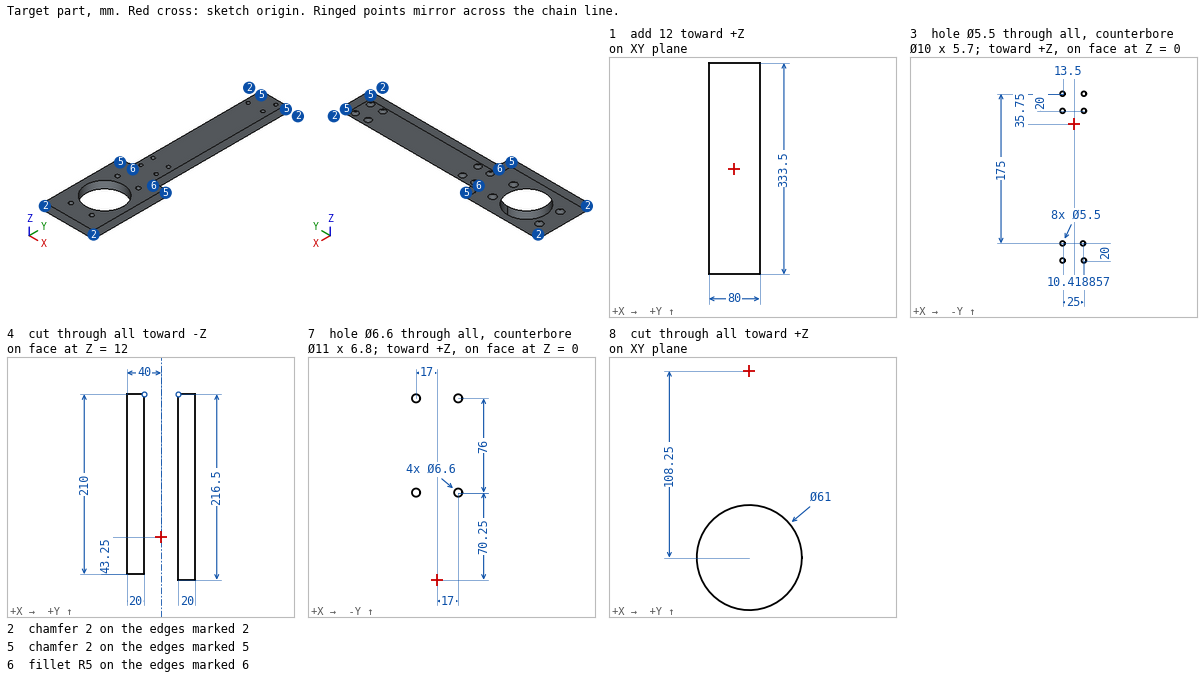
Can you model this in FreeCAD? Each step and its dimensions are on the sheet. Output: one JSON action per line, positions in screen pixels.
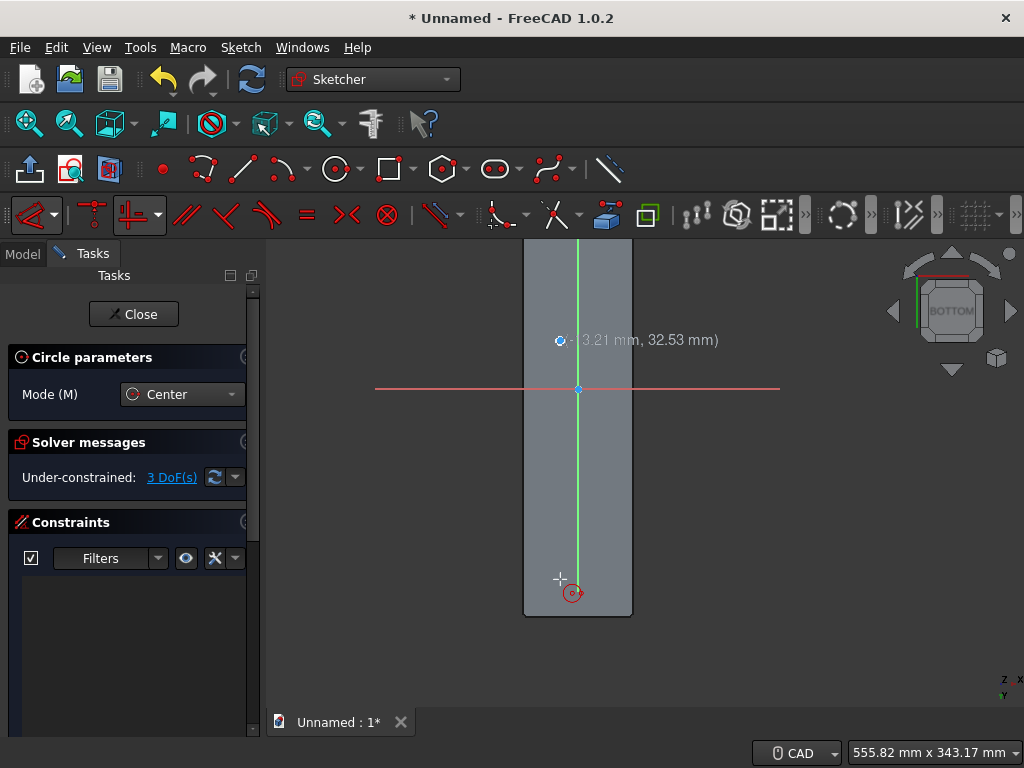
{"action": "left_click", "coordinate": [560, 579]}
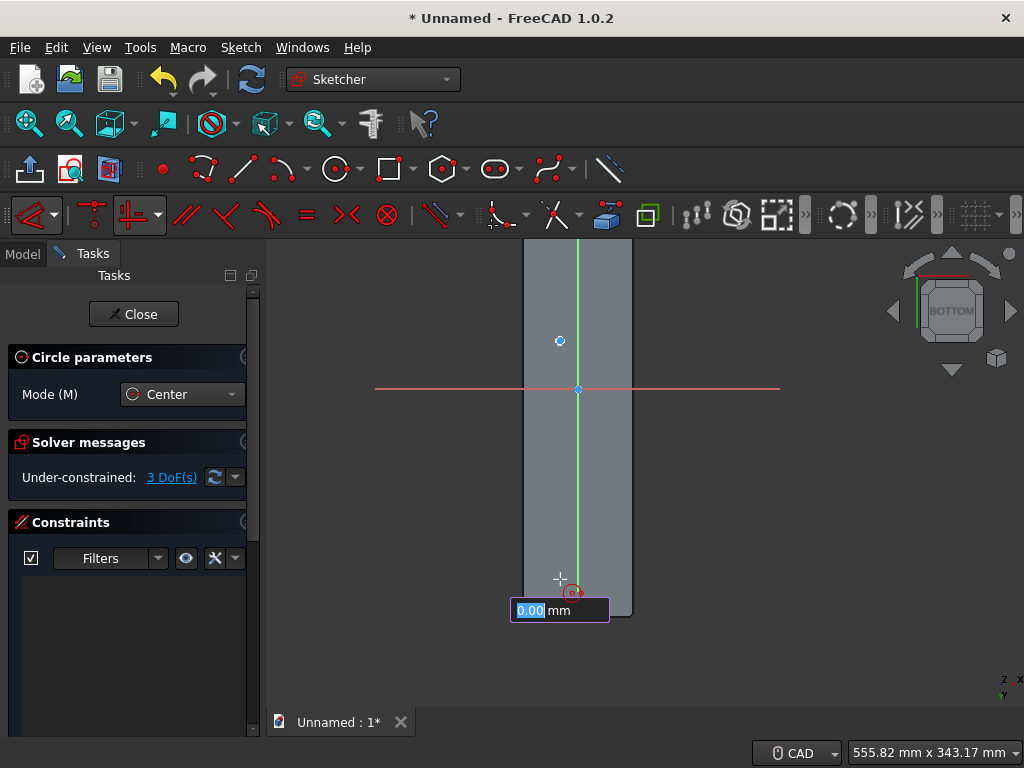
{"action": "scroll", "coordinate": [562, 576], "scroll_direction": "up", "scroll_amount": 8}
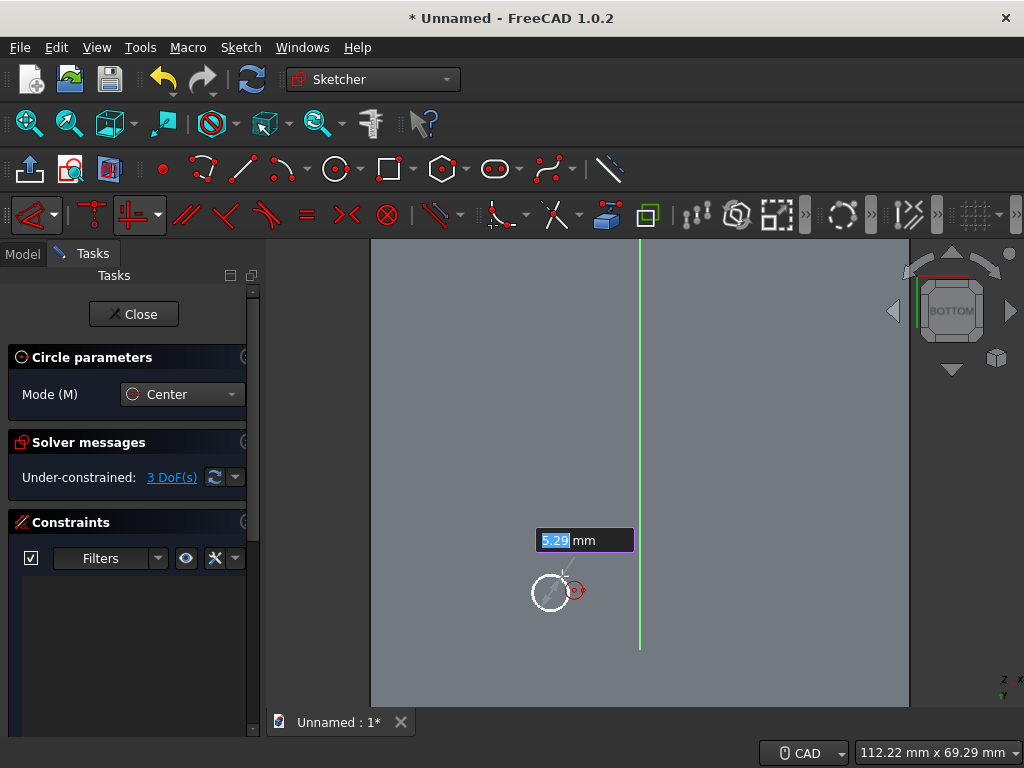
{"action": "left_click", "coordinate": [562, 575]}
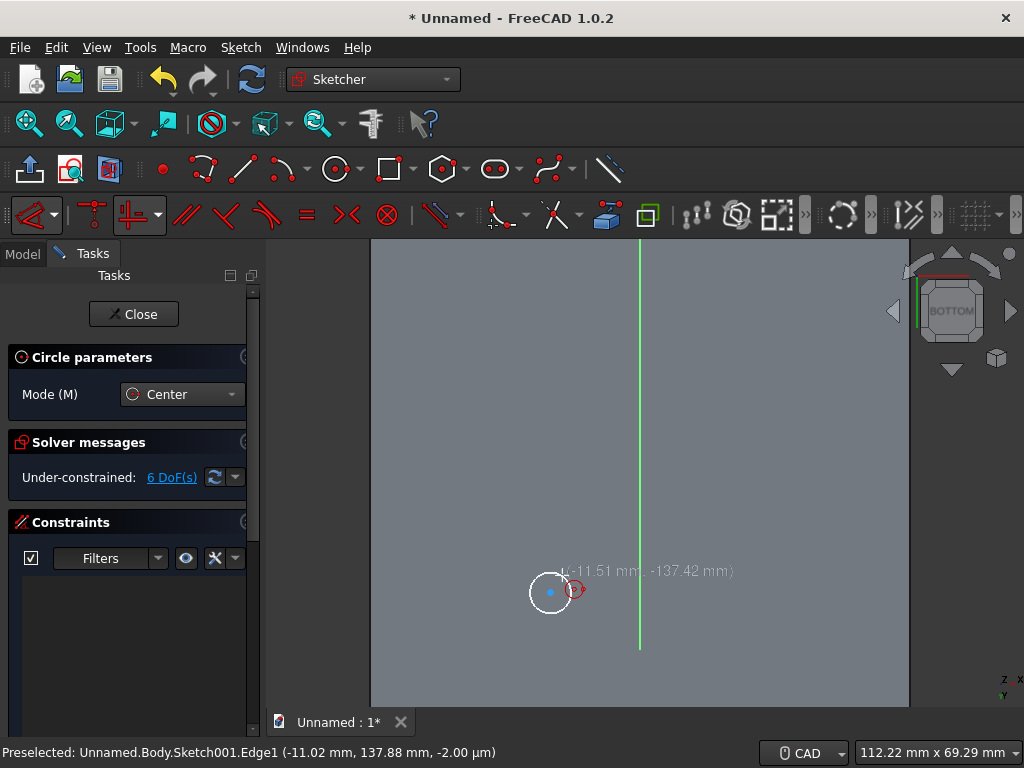
{"action": "scroll", "coordinate": [562, 576], "scroll_direction": "down", "scroll_amount": 8}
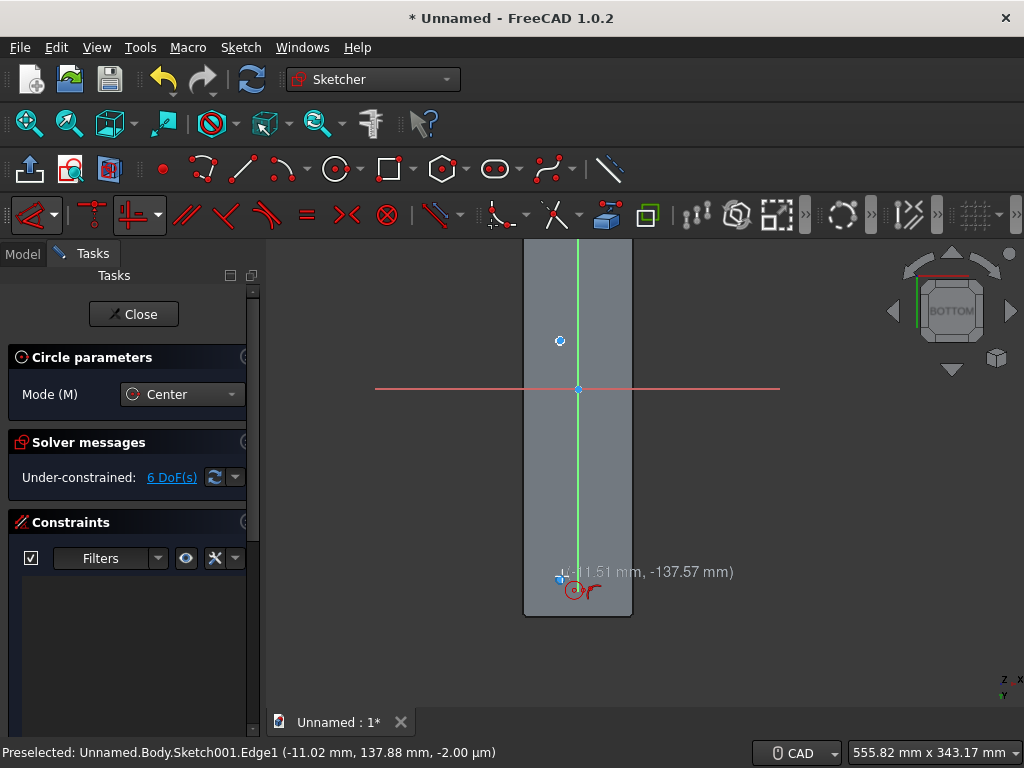
{"action": "scroll", "coordinate": [594, 606], "scroll_direction": "up", "scroll_amount": 9}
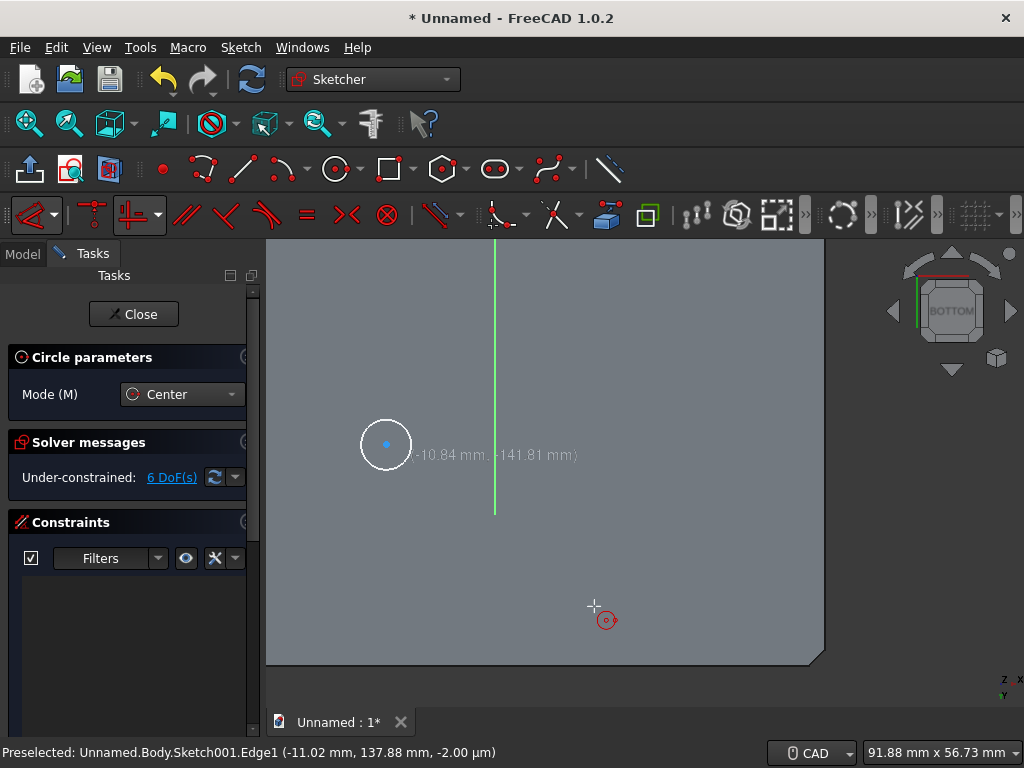
{"action": "scroll", "coordinate": [594, 606], "scroll_direction": "down", "scroll_amount": 9}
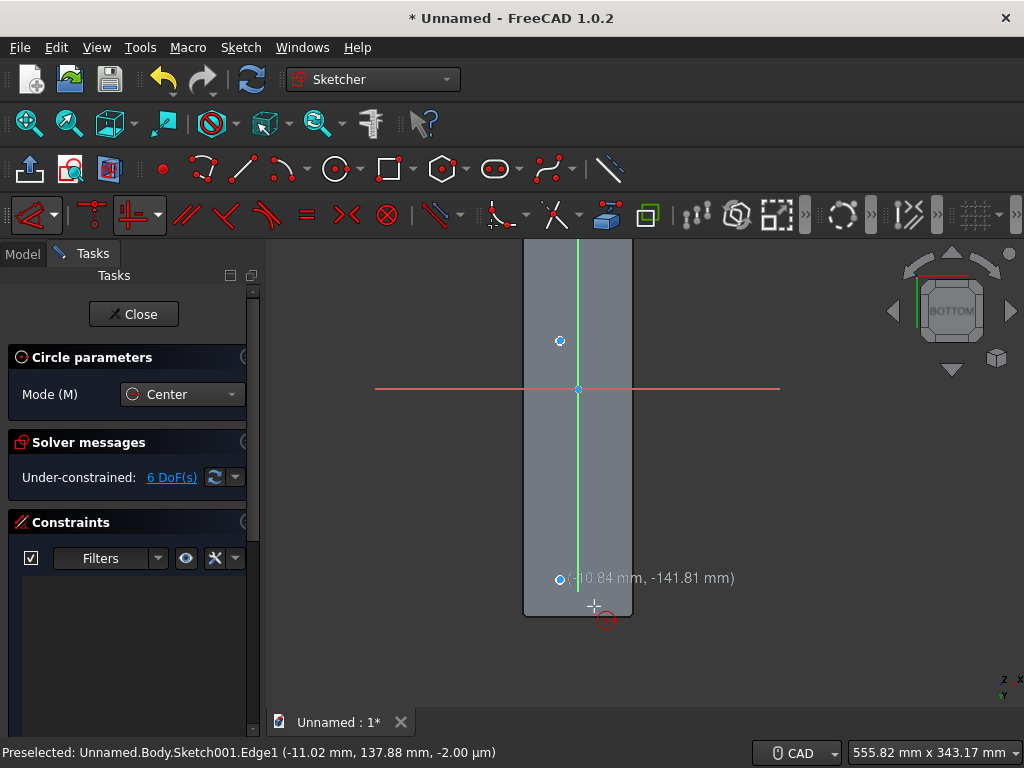
{"action": "left_click", "coordinate": [594, 606]}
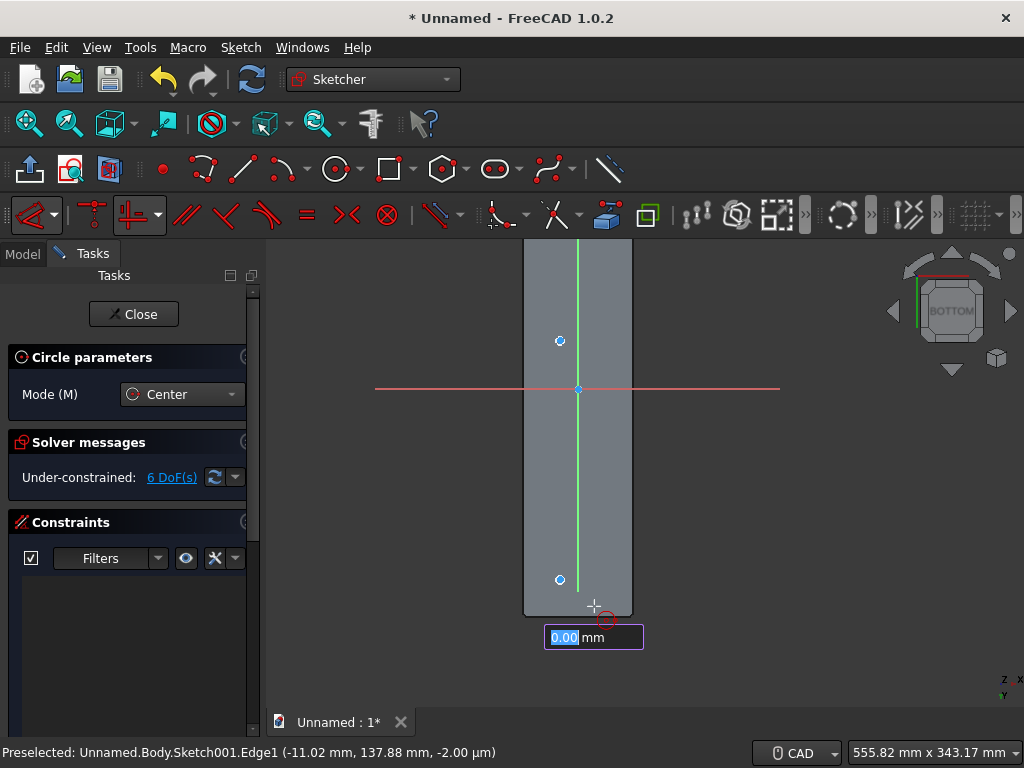
{"action": "scroll", "coordinate": [596, 604], "scroll_direction": "up", "scroll_amount": 8}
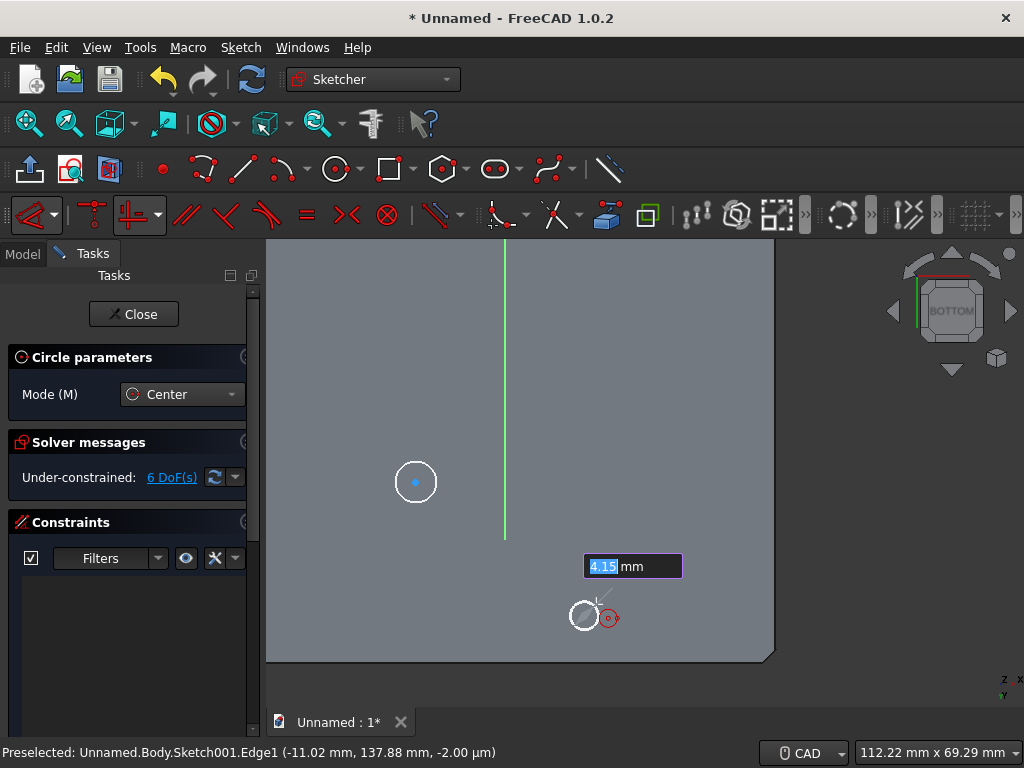
{"action": "left_click", "coordinate": [596, 599]}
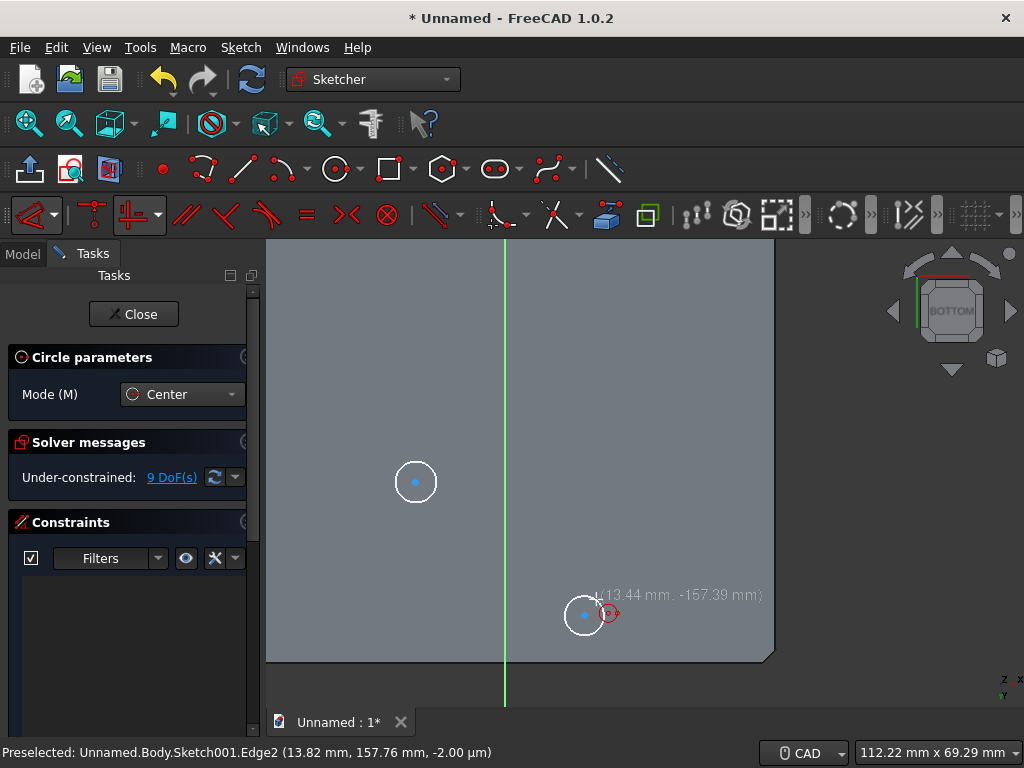
{"action": "scroll", "coordinate": [596, 604], "scroll_direction": "down", "scroll_amount": 8}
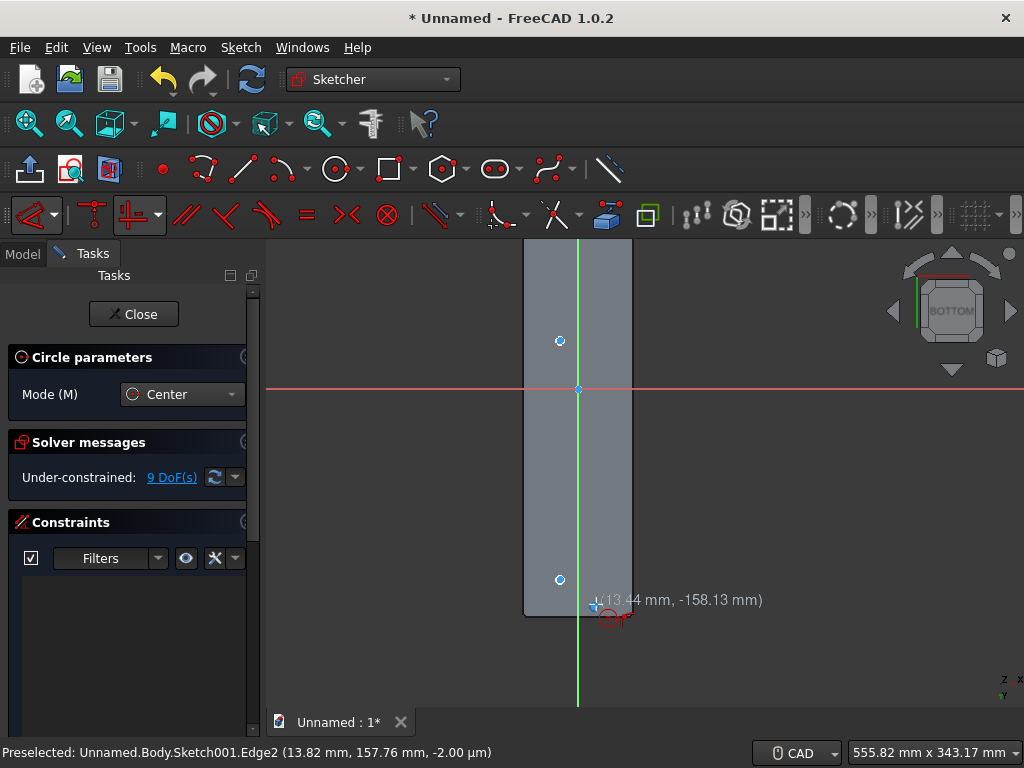
{"action": "left_click", "coordinate": [592, 579]}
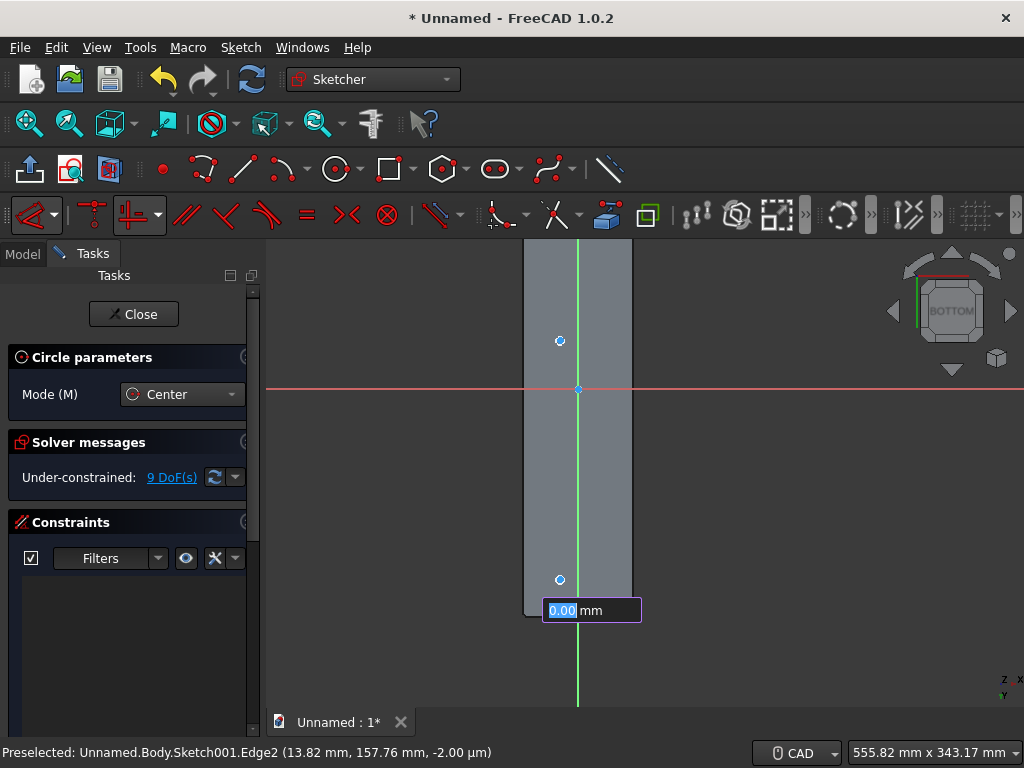
{"action": "scroll", "coordinate": [595, 576], "scroll_direction": "up", "scroll_amount": 8}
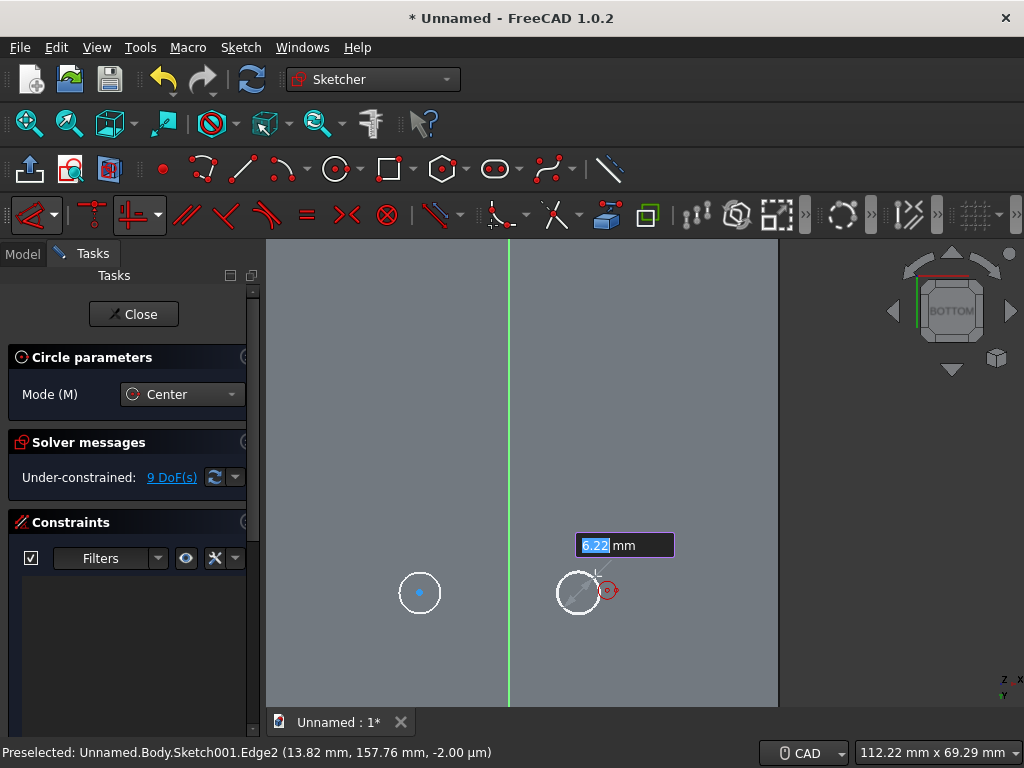
{"action": "left_click", "coordinate": [593, 575]}